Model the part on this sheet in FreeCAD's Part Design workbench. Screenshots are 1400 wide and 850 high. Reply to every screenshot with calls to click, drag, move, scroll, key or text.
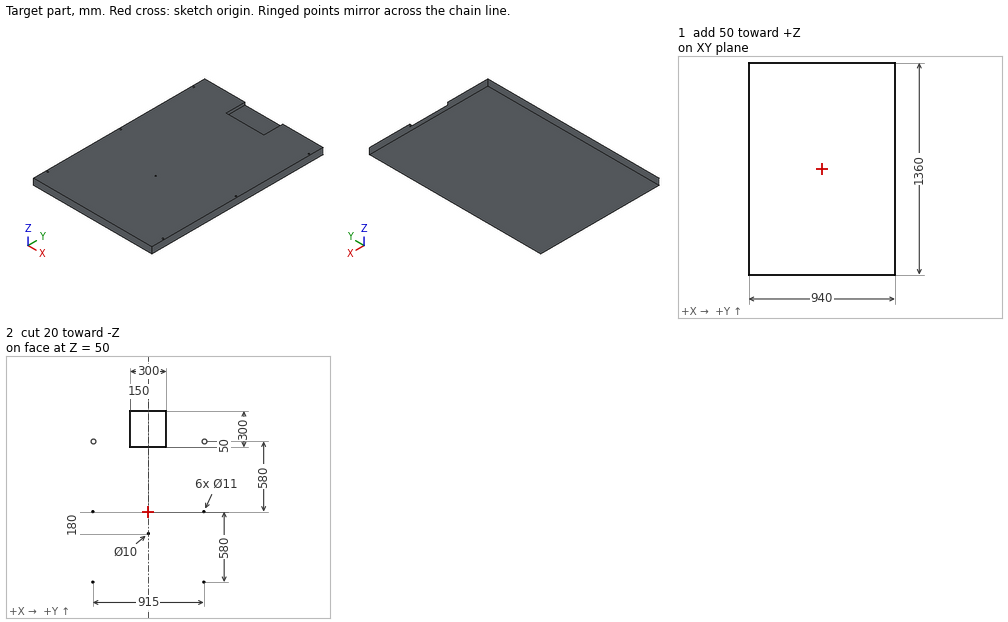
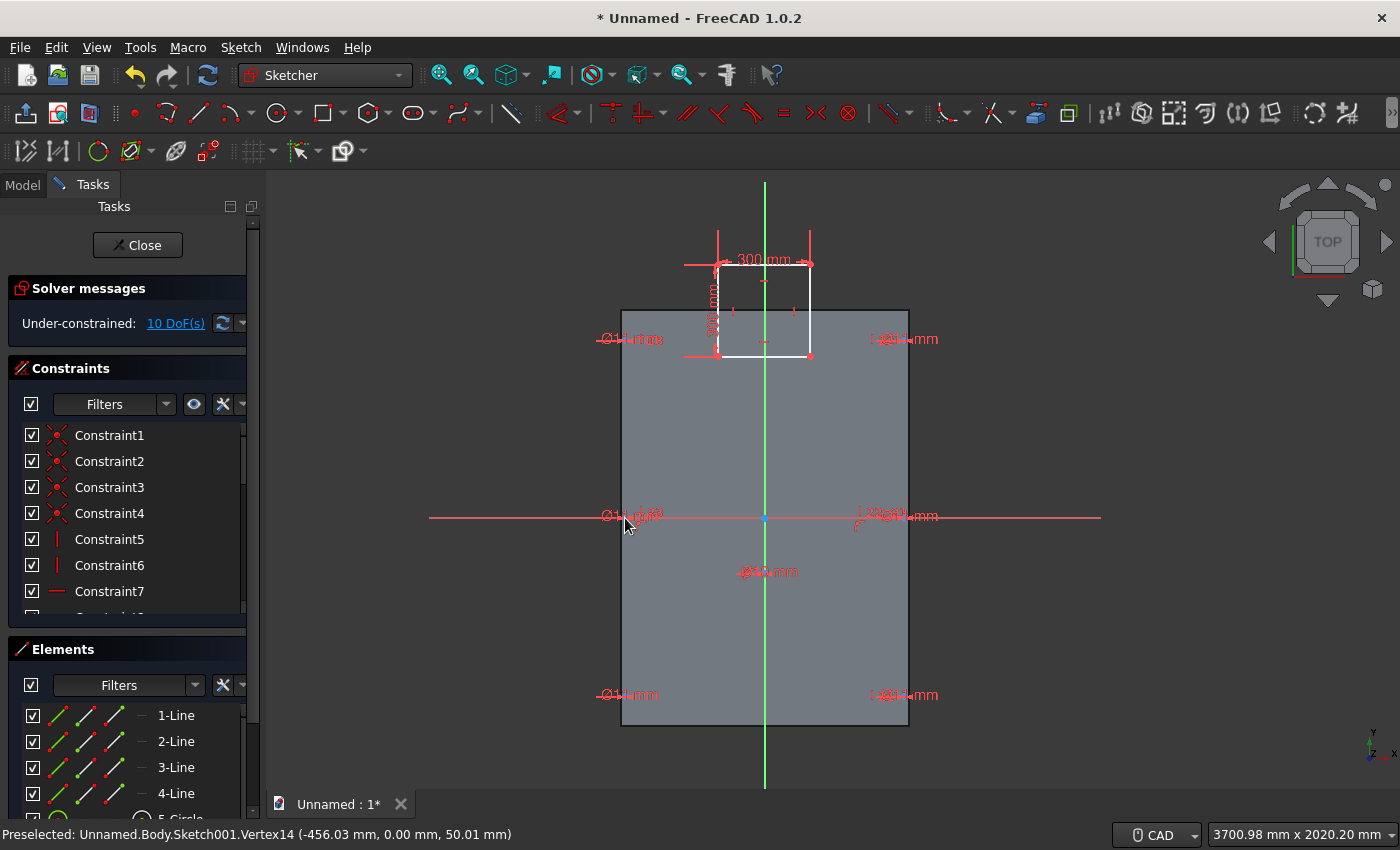
click(625, 518)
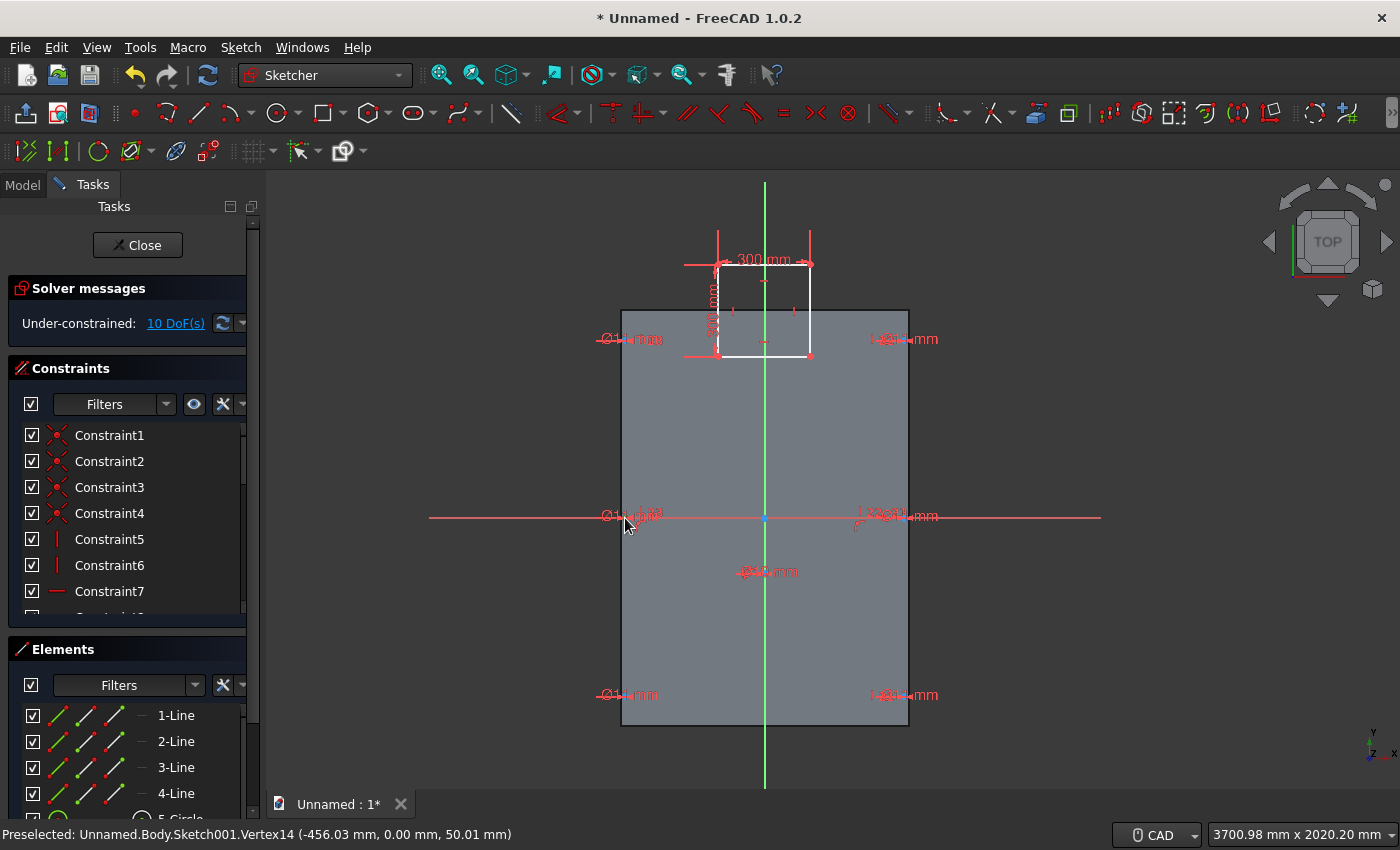
click(625, 697)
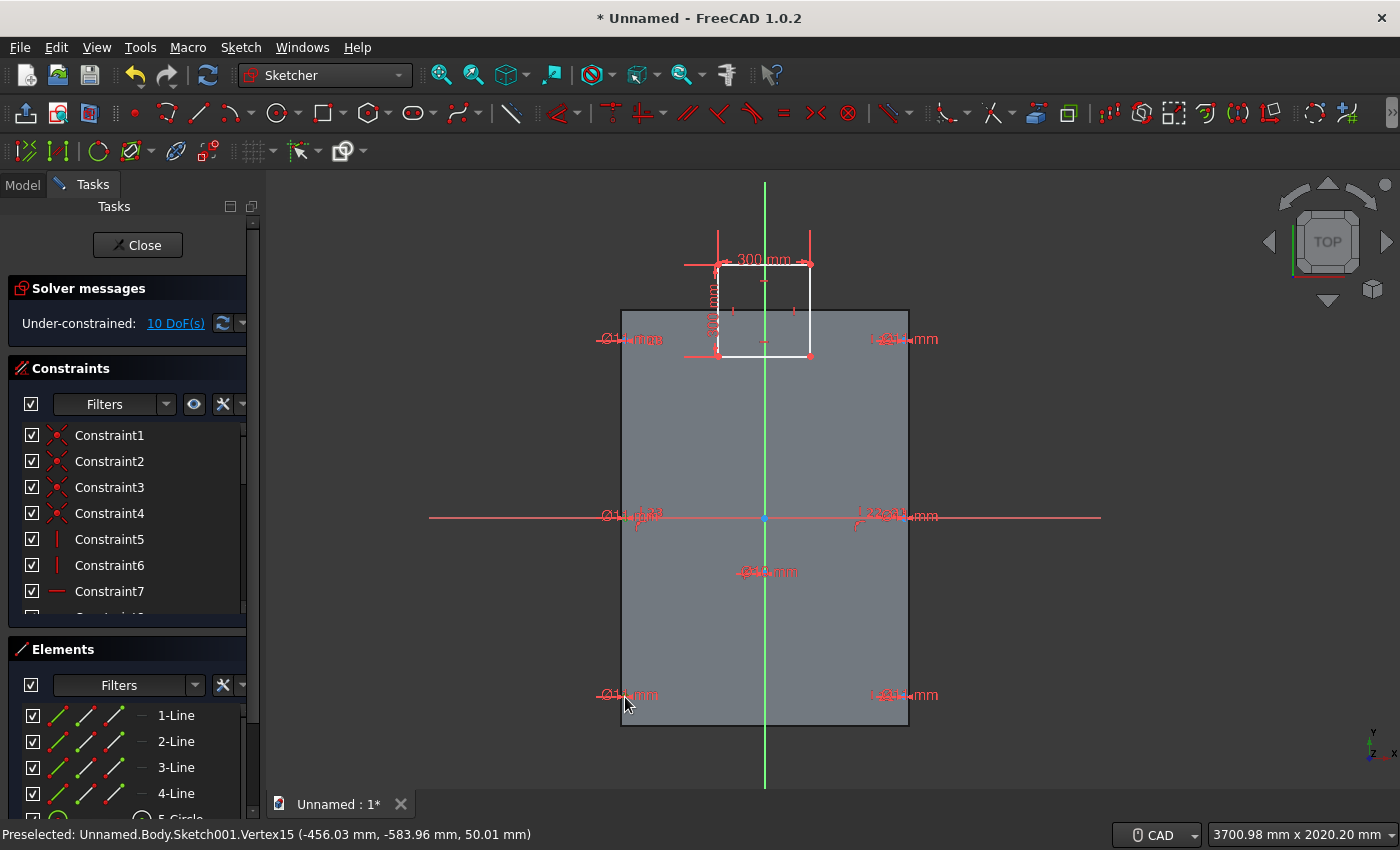
click(666, 114)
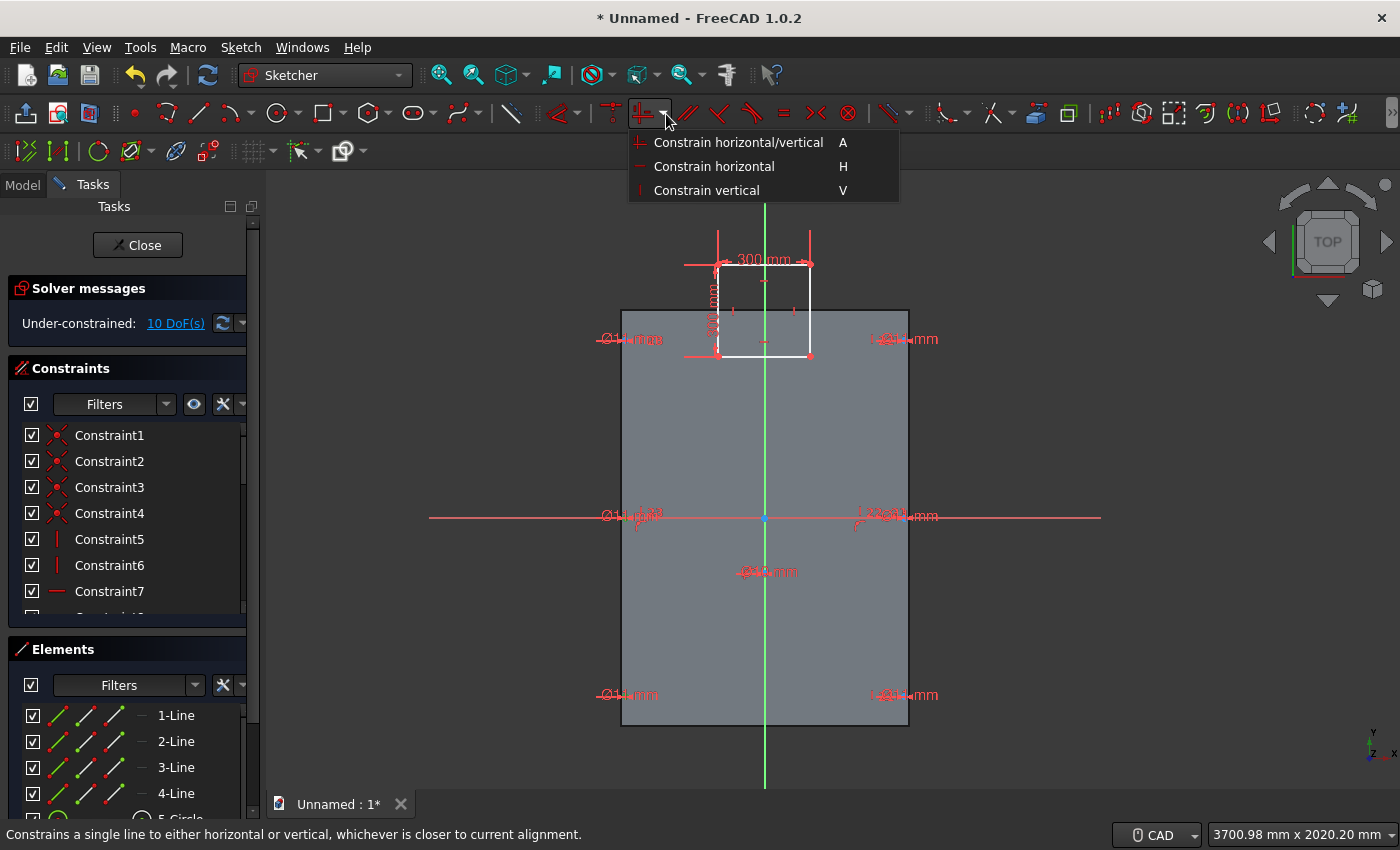
click(764, 190)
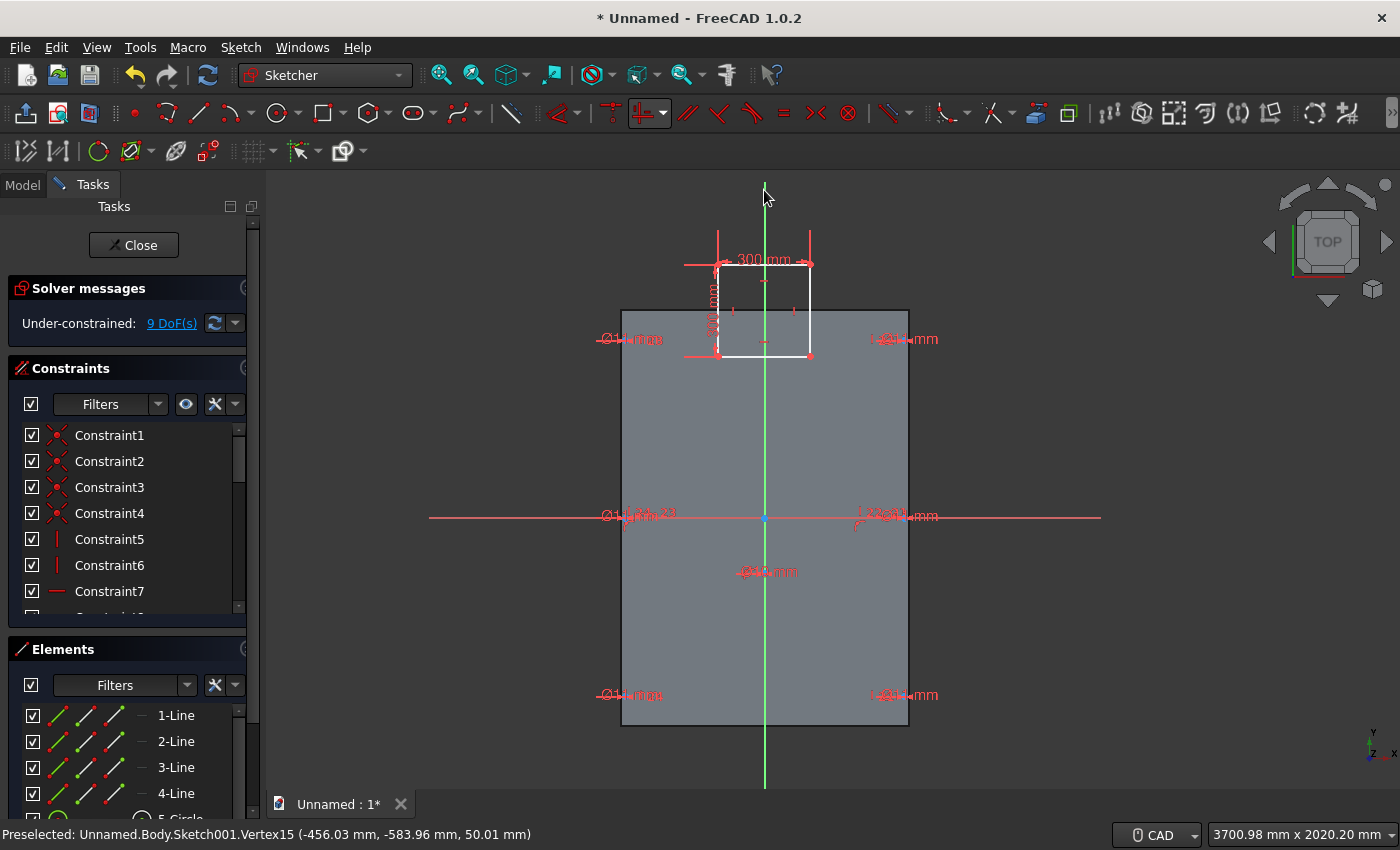
click(905, 697)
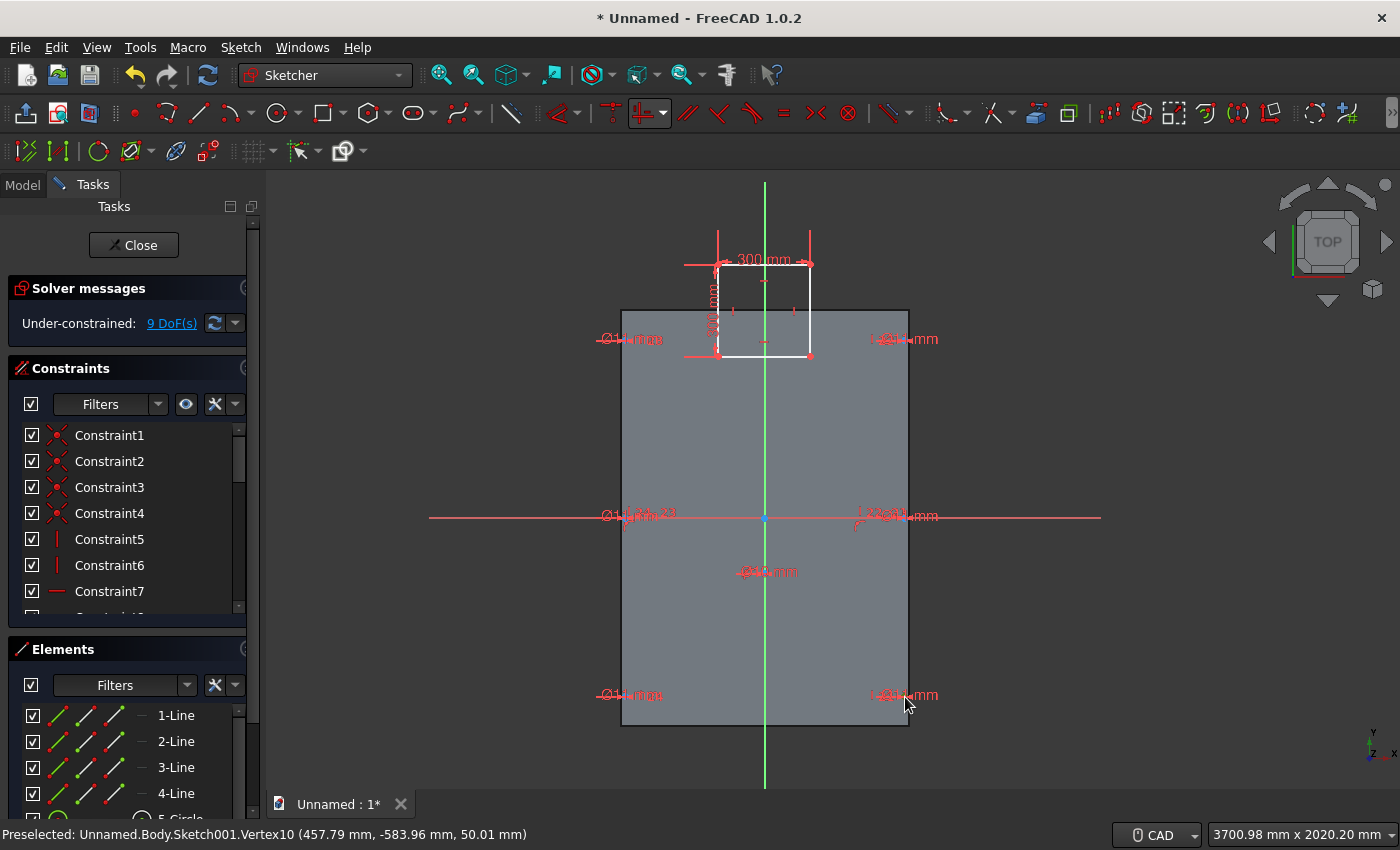
click(625, 697)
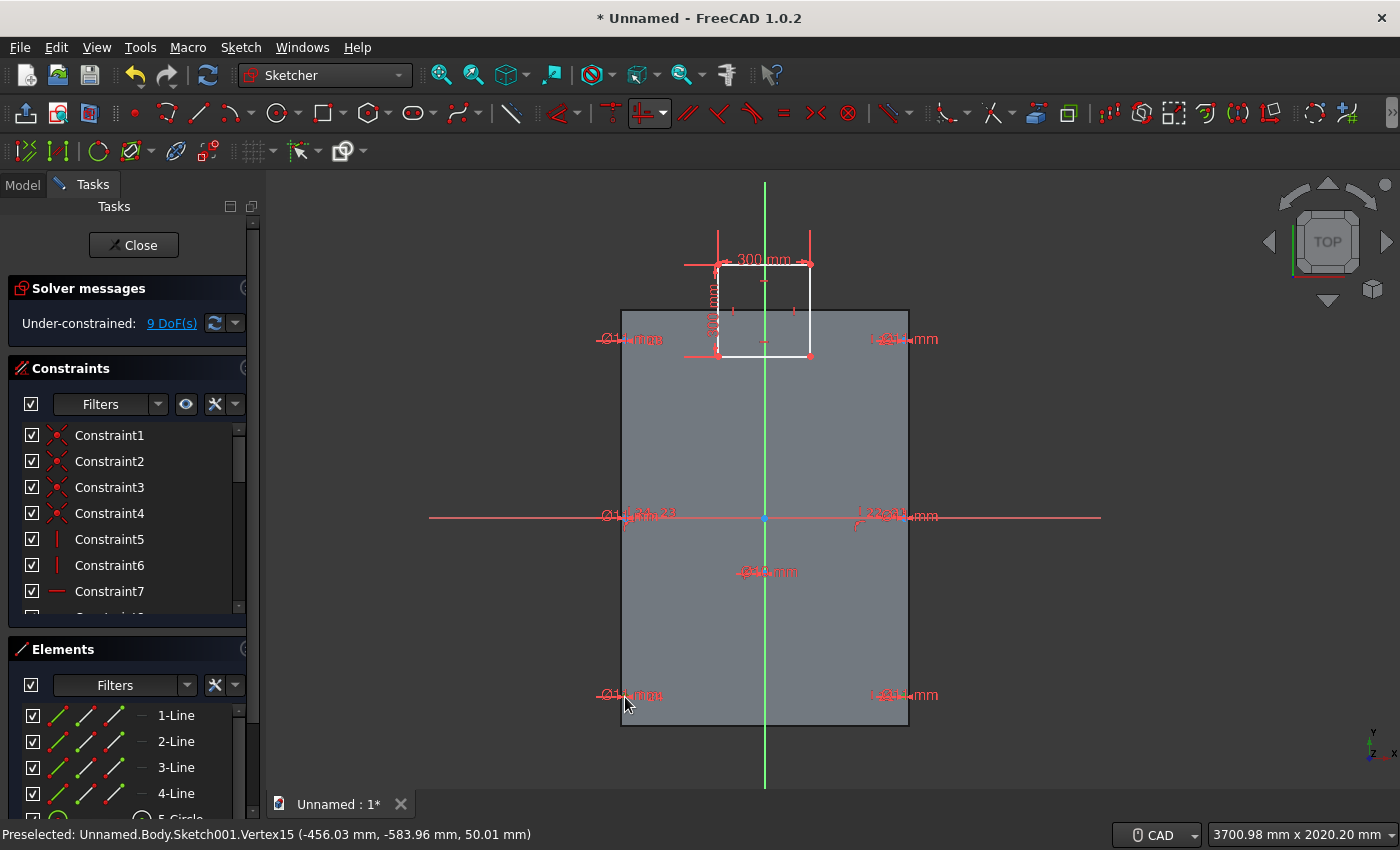
key(h)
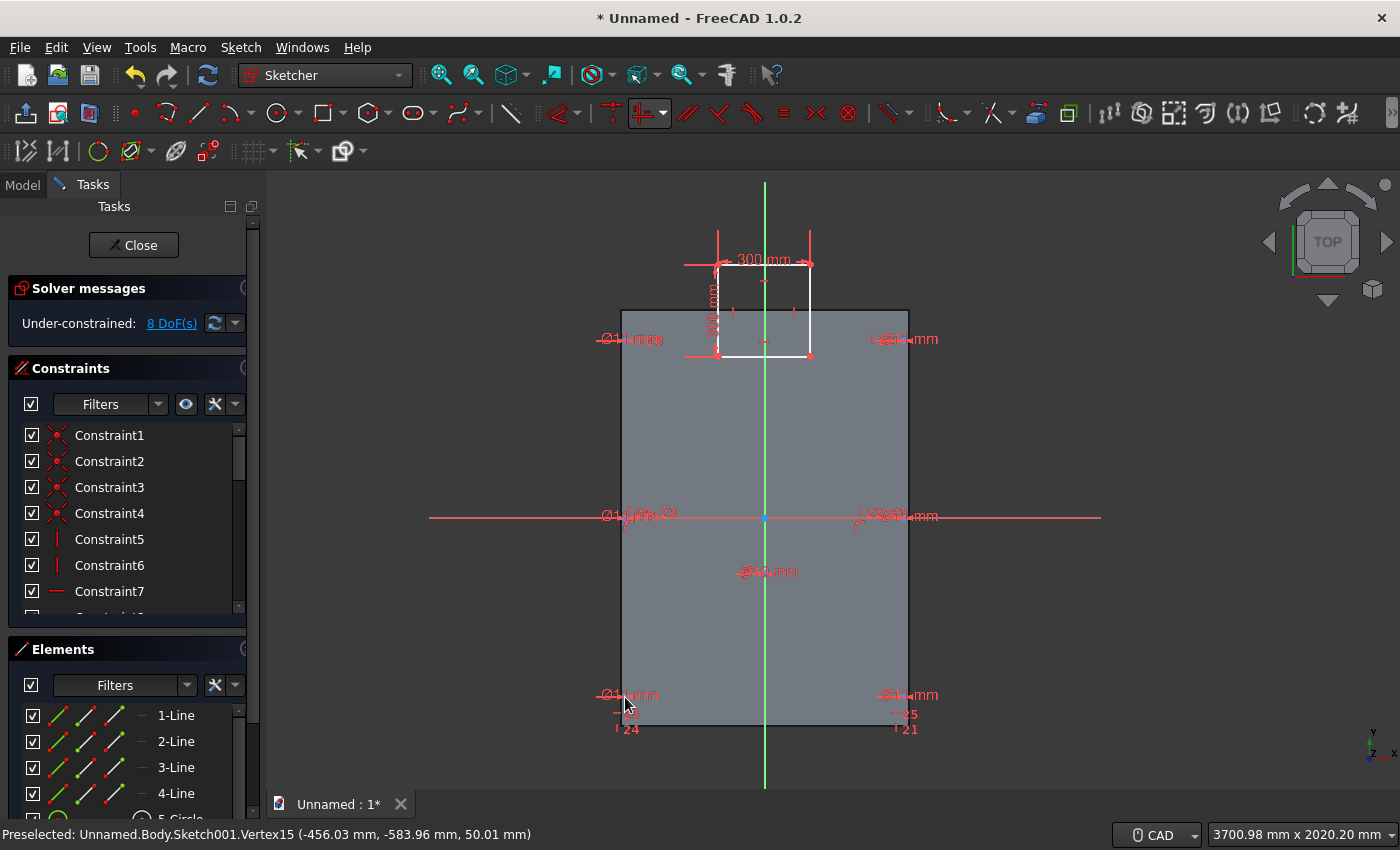
click(905, 341)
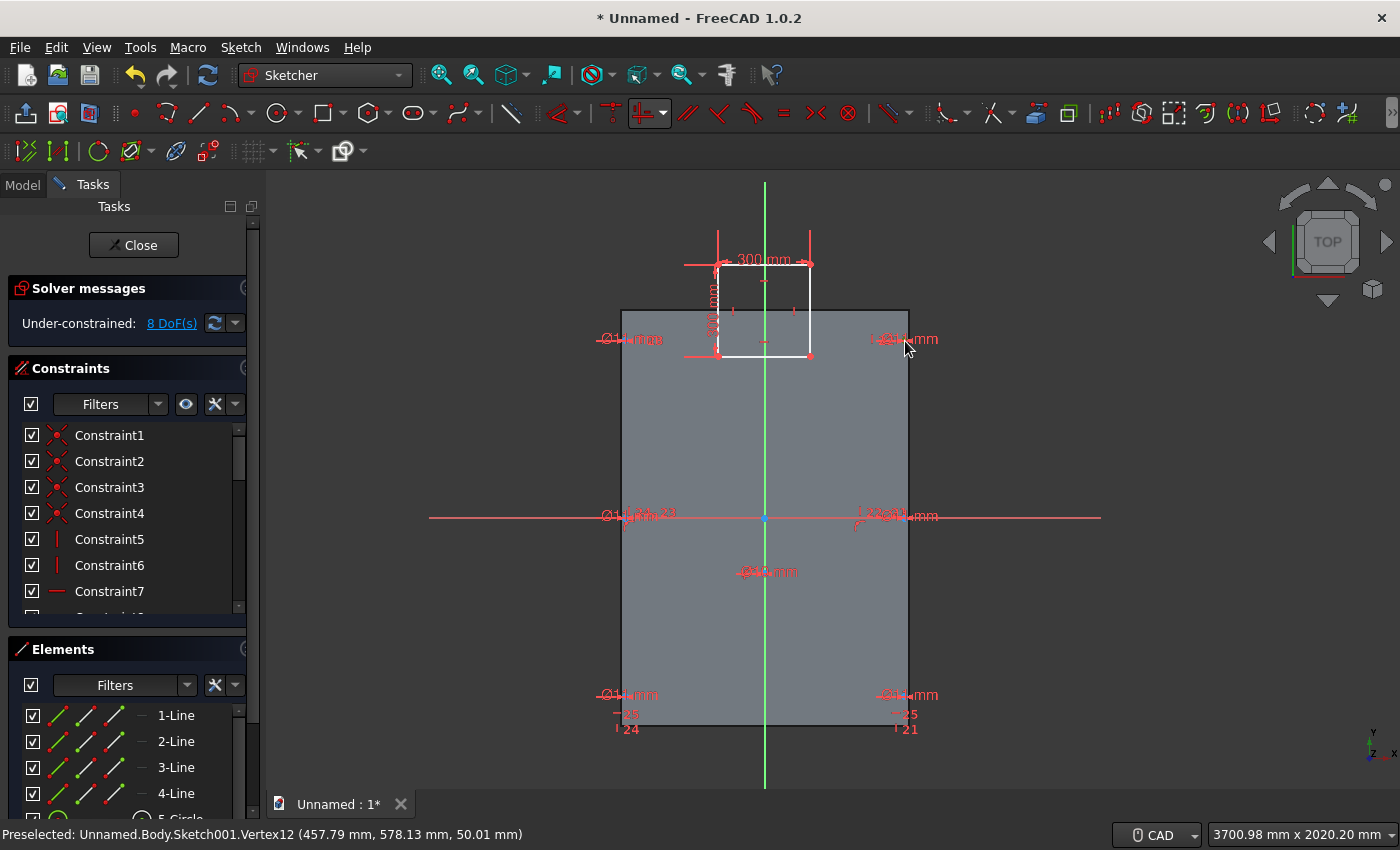
click(625, 341)